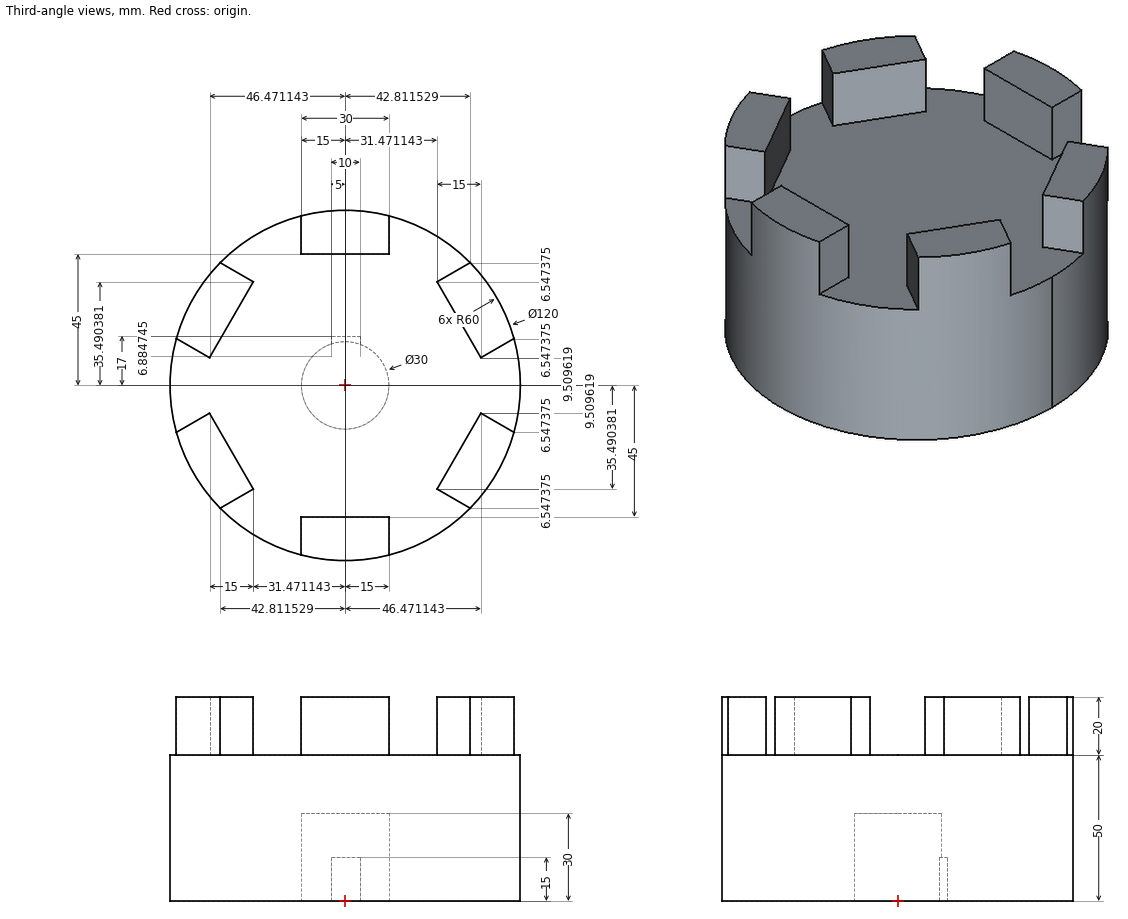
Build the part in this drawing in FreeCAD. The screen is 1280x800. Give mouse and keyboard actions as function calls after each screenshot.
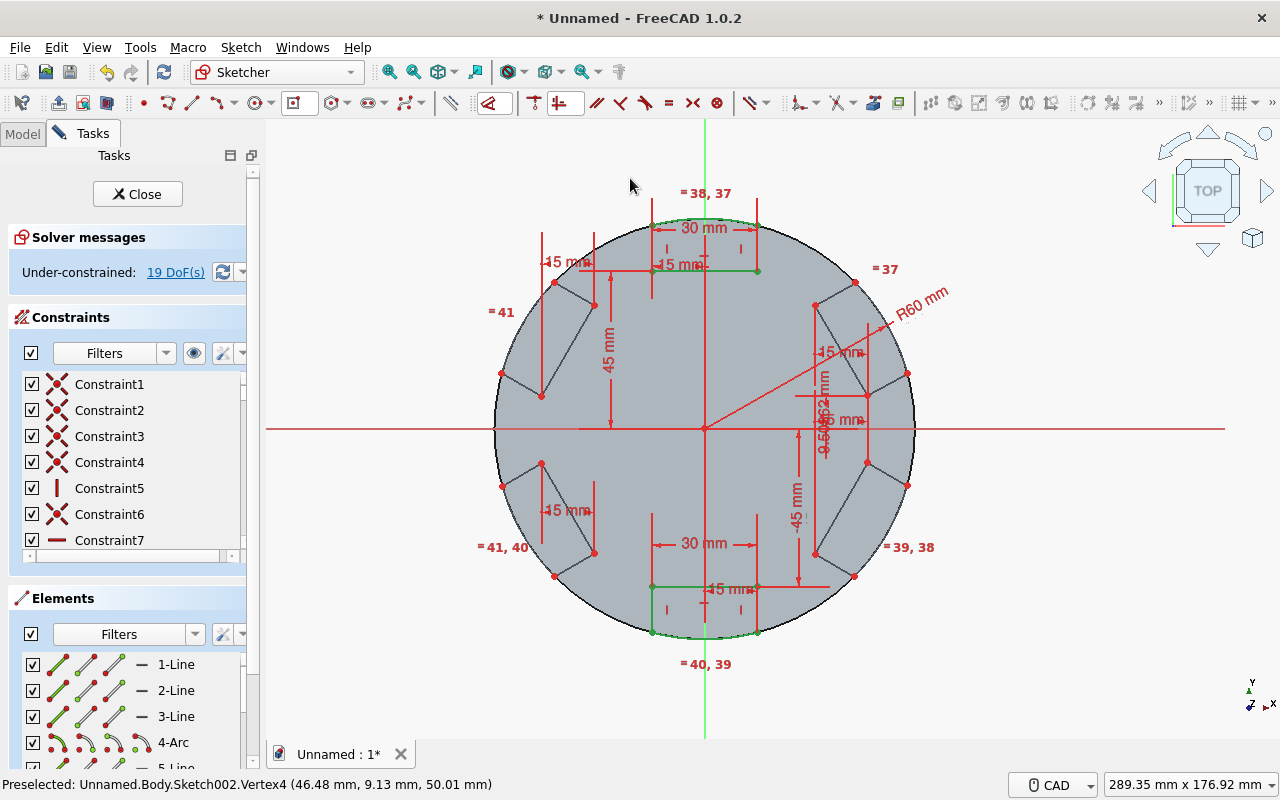
click(868, 463)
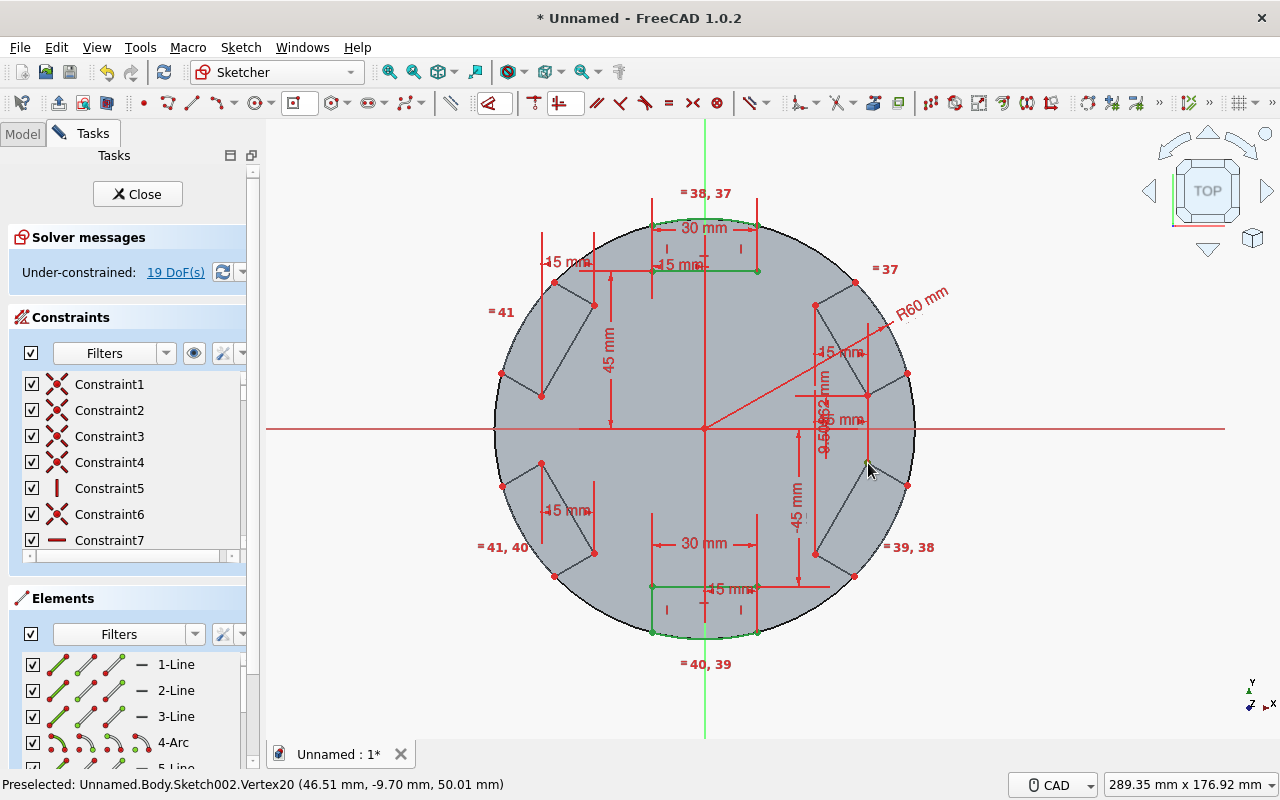
key(i)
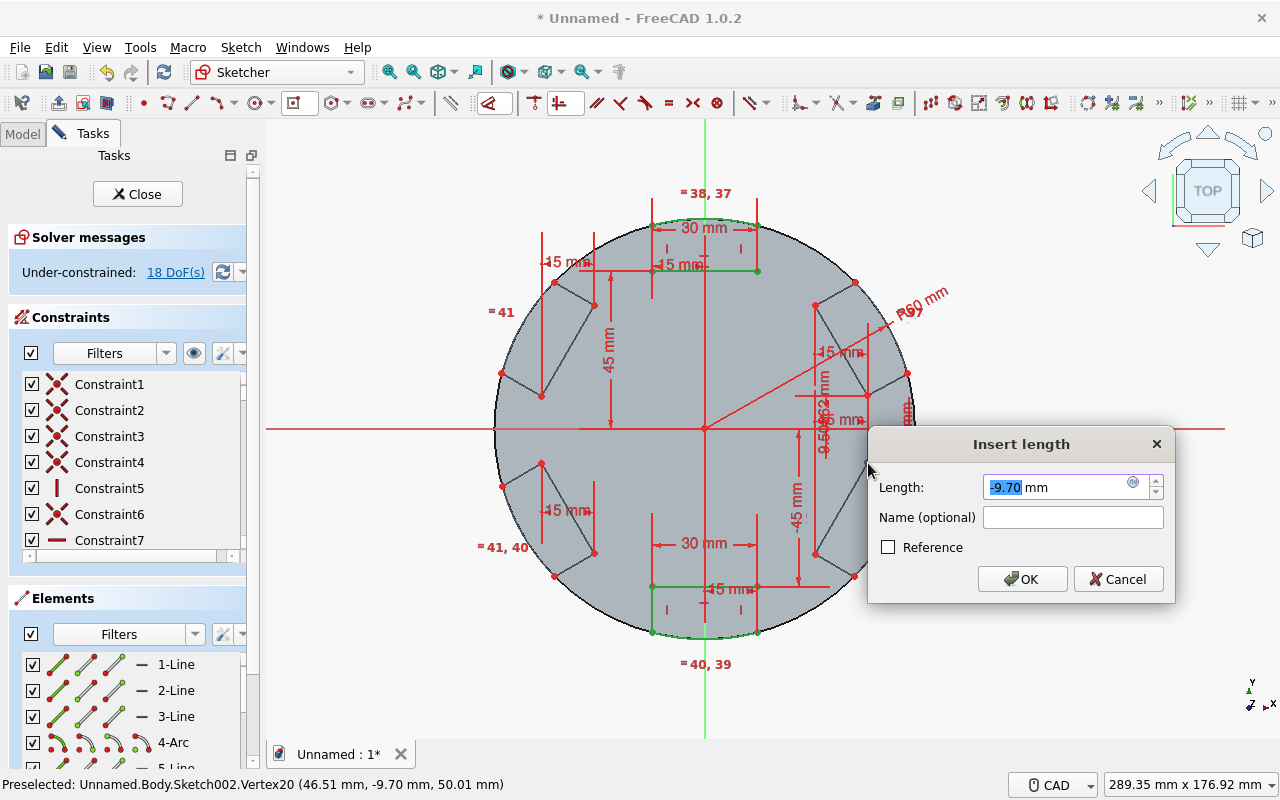
text(-9.509619)
key(Return)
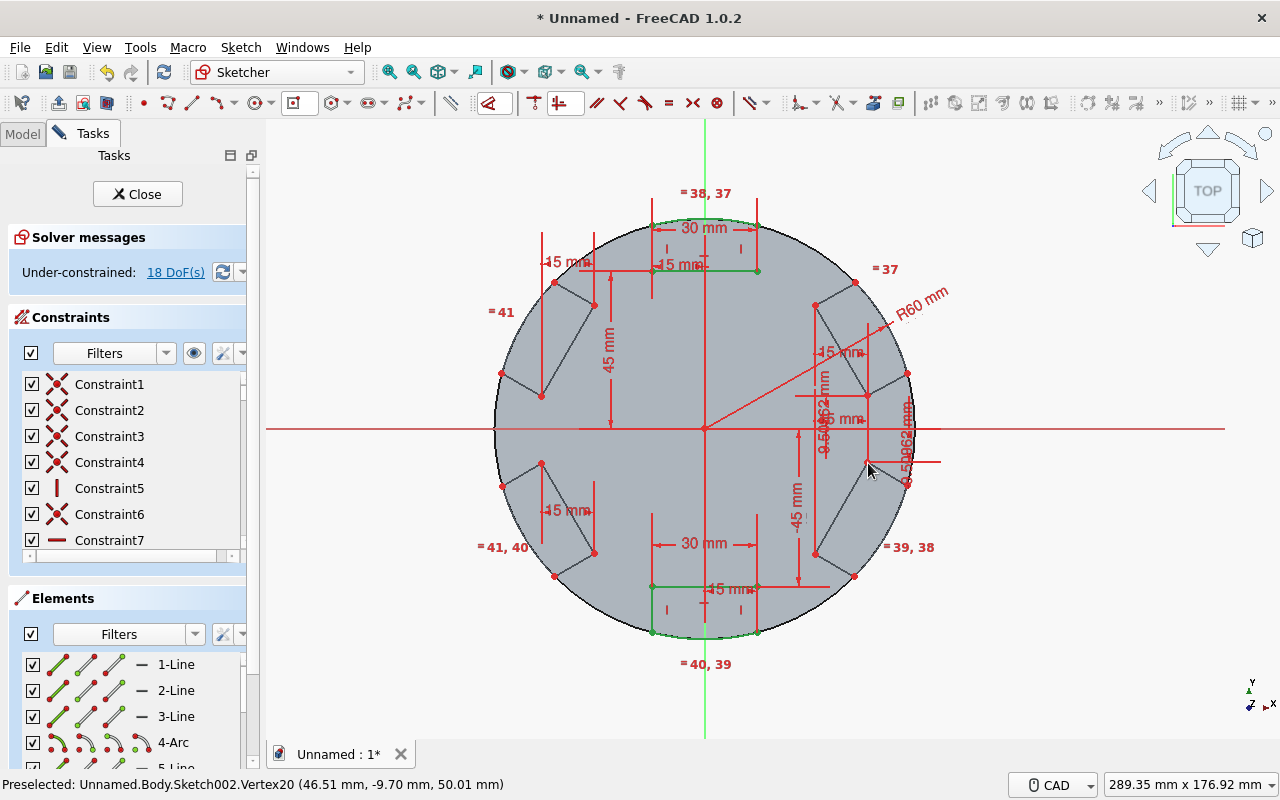
click(542, 463)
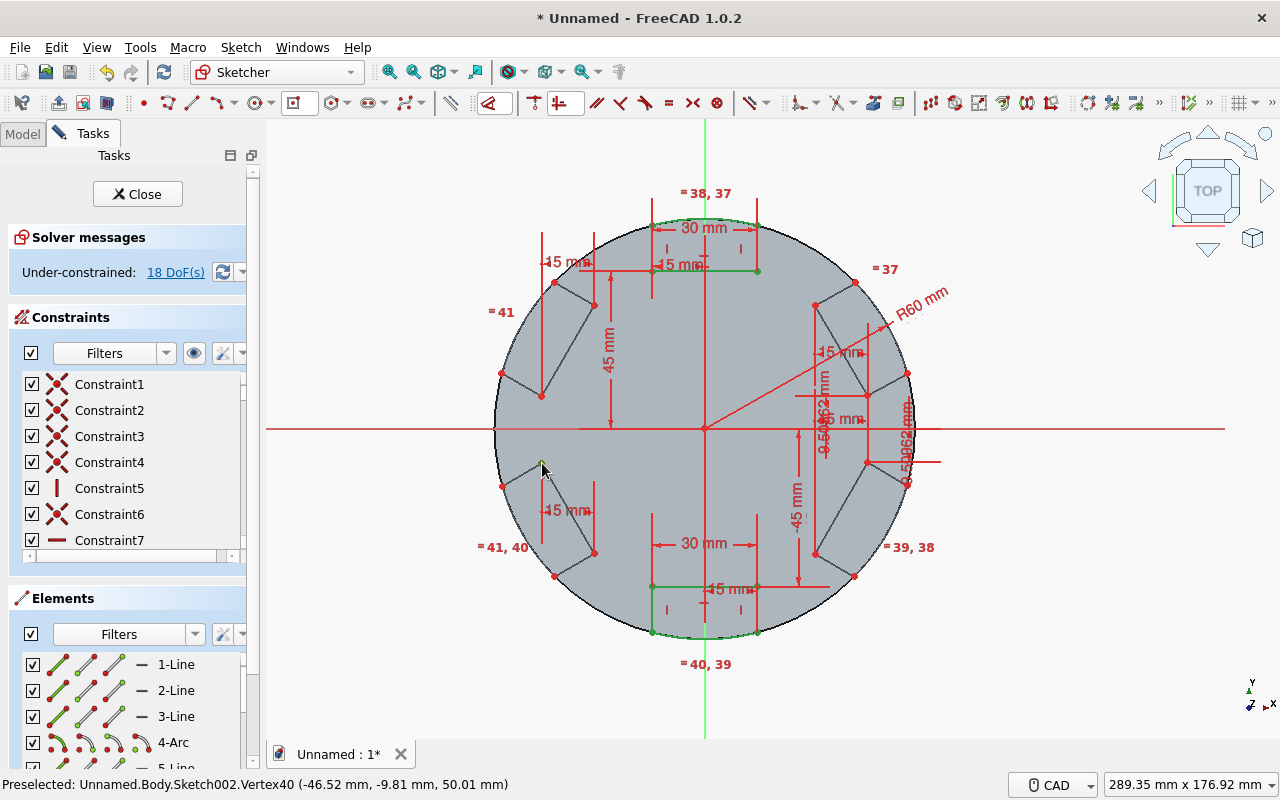
key(i)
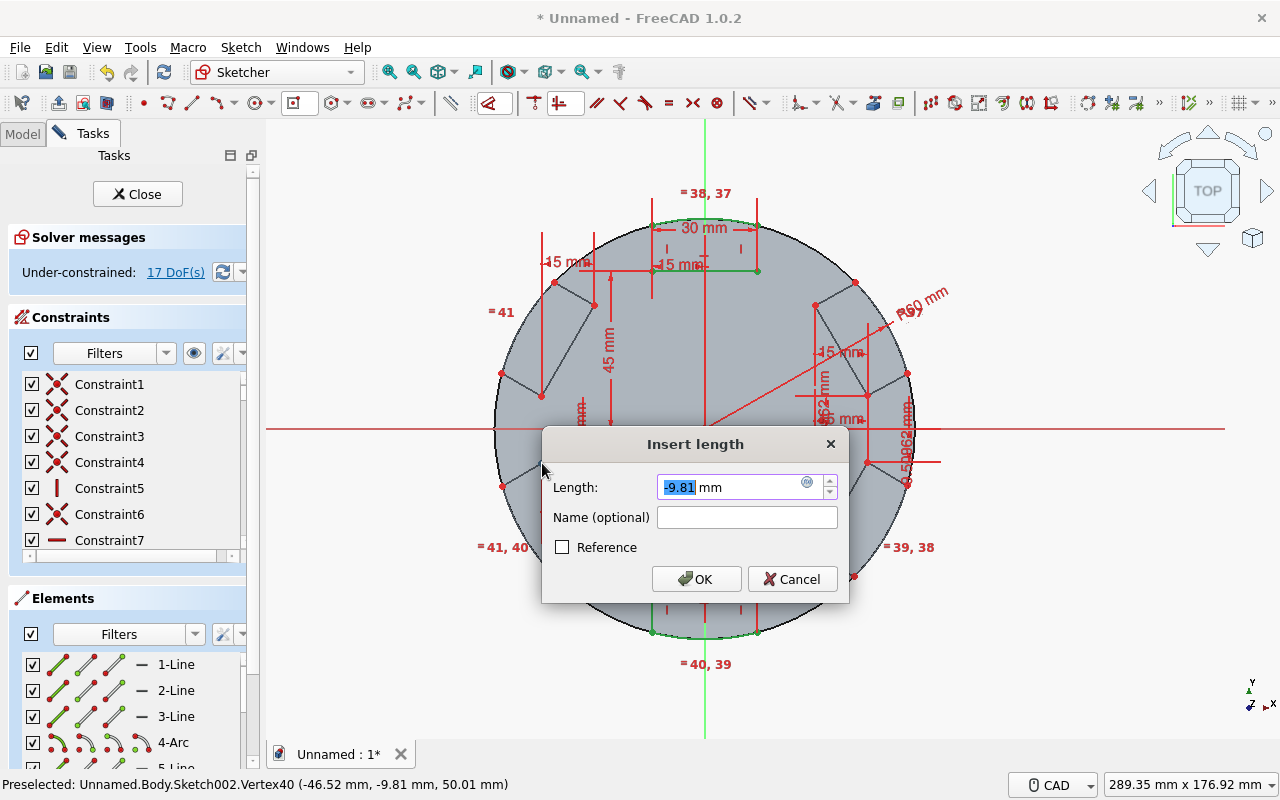
text(-9.509619)
key(Return)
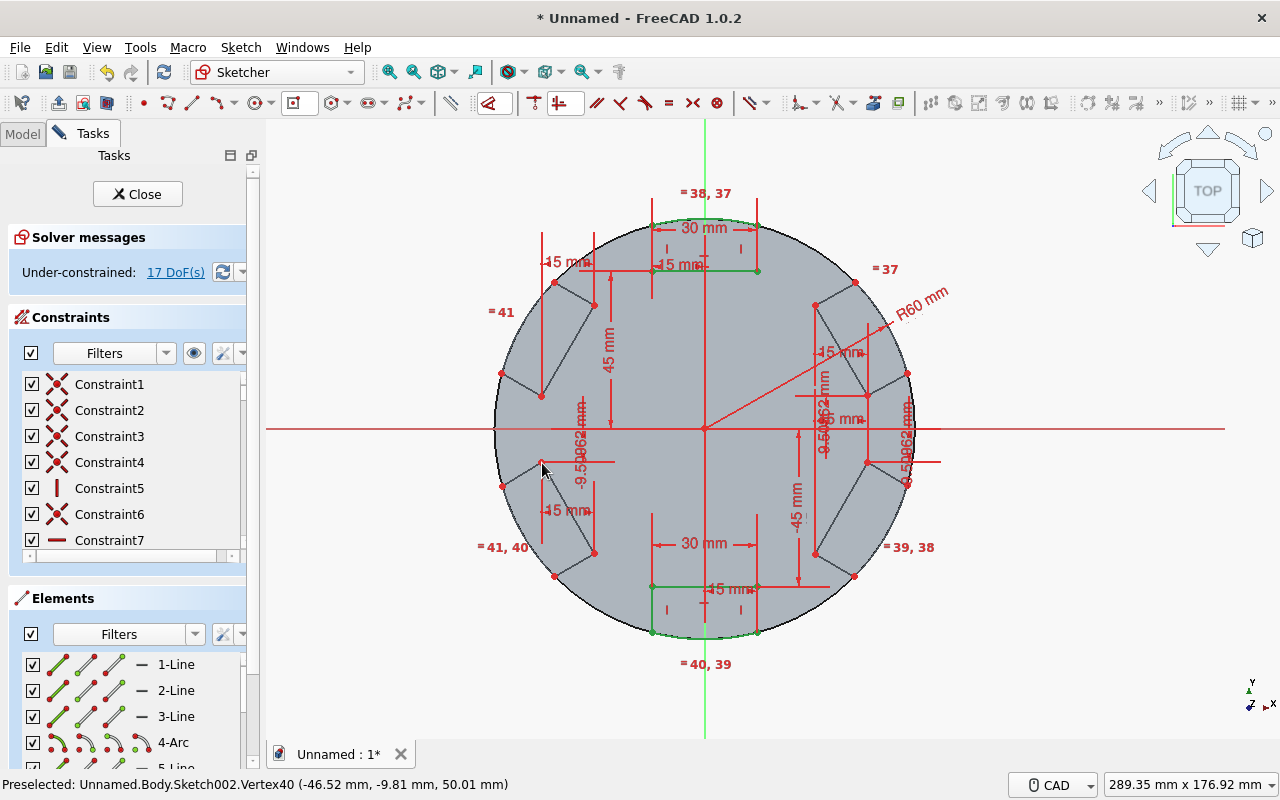
click(542, 396)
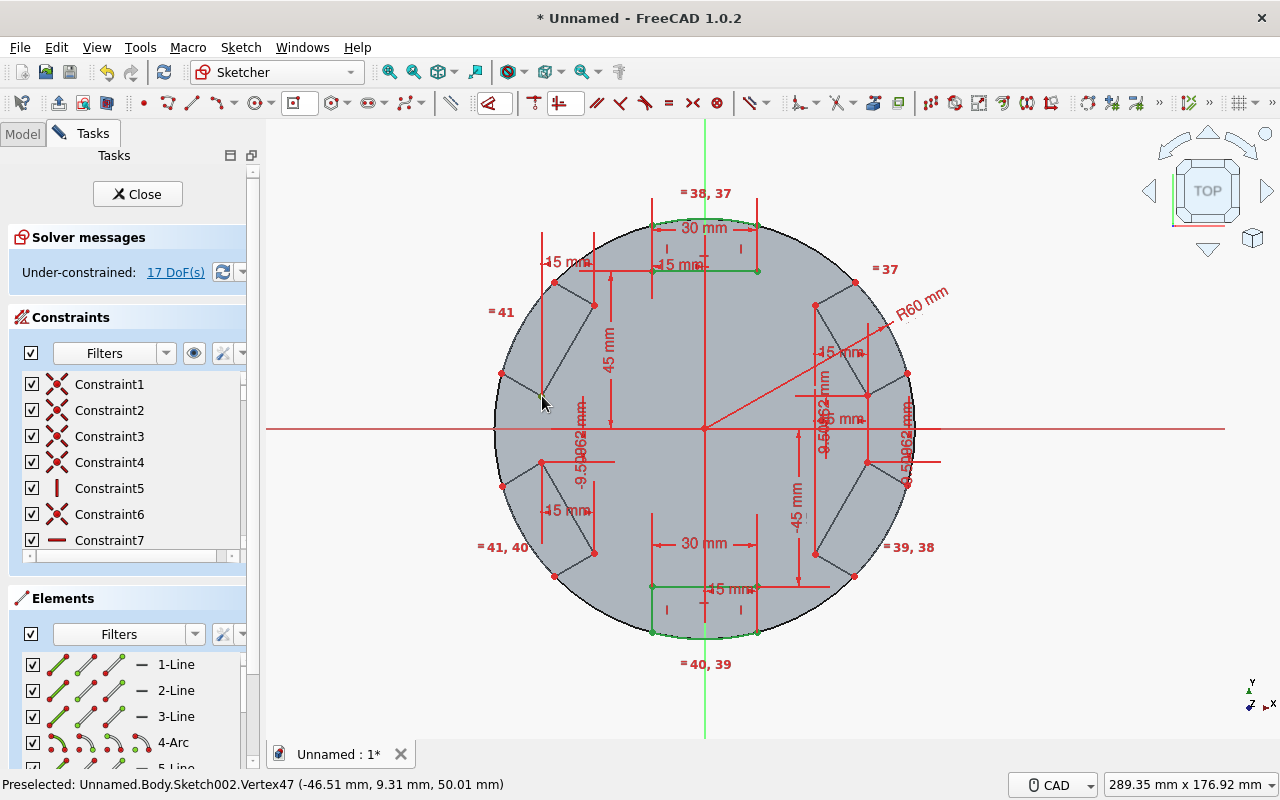
click(506, 104)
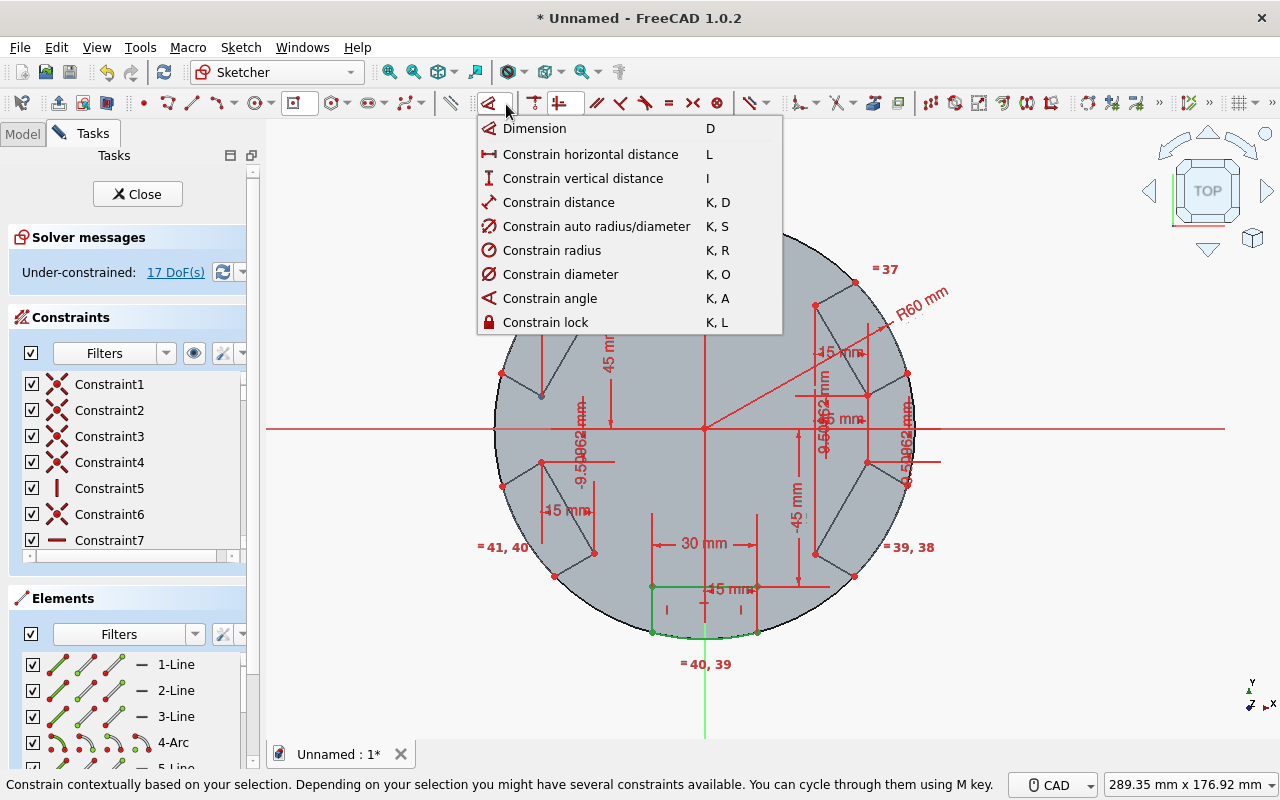
click(630, 178)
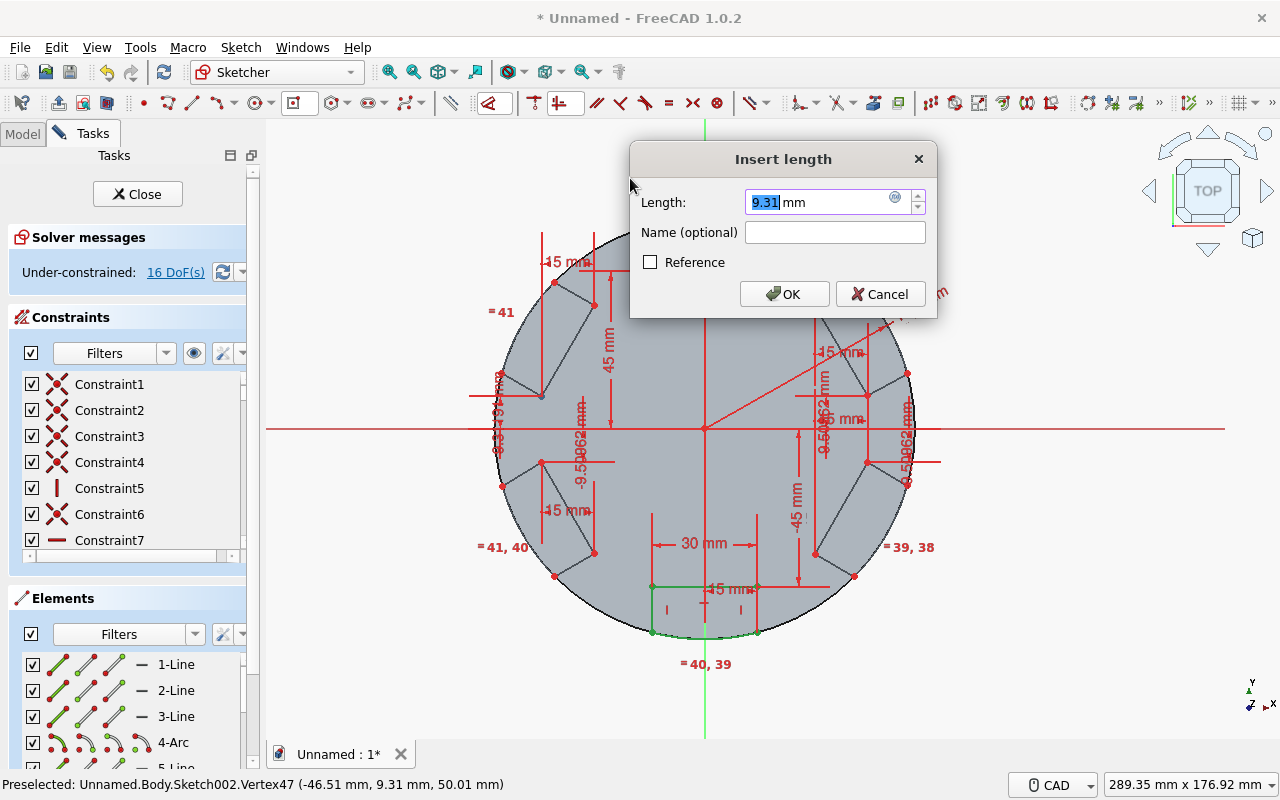
text(9.509619)
key(Return)